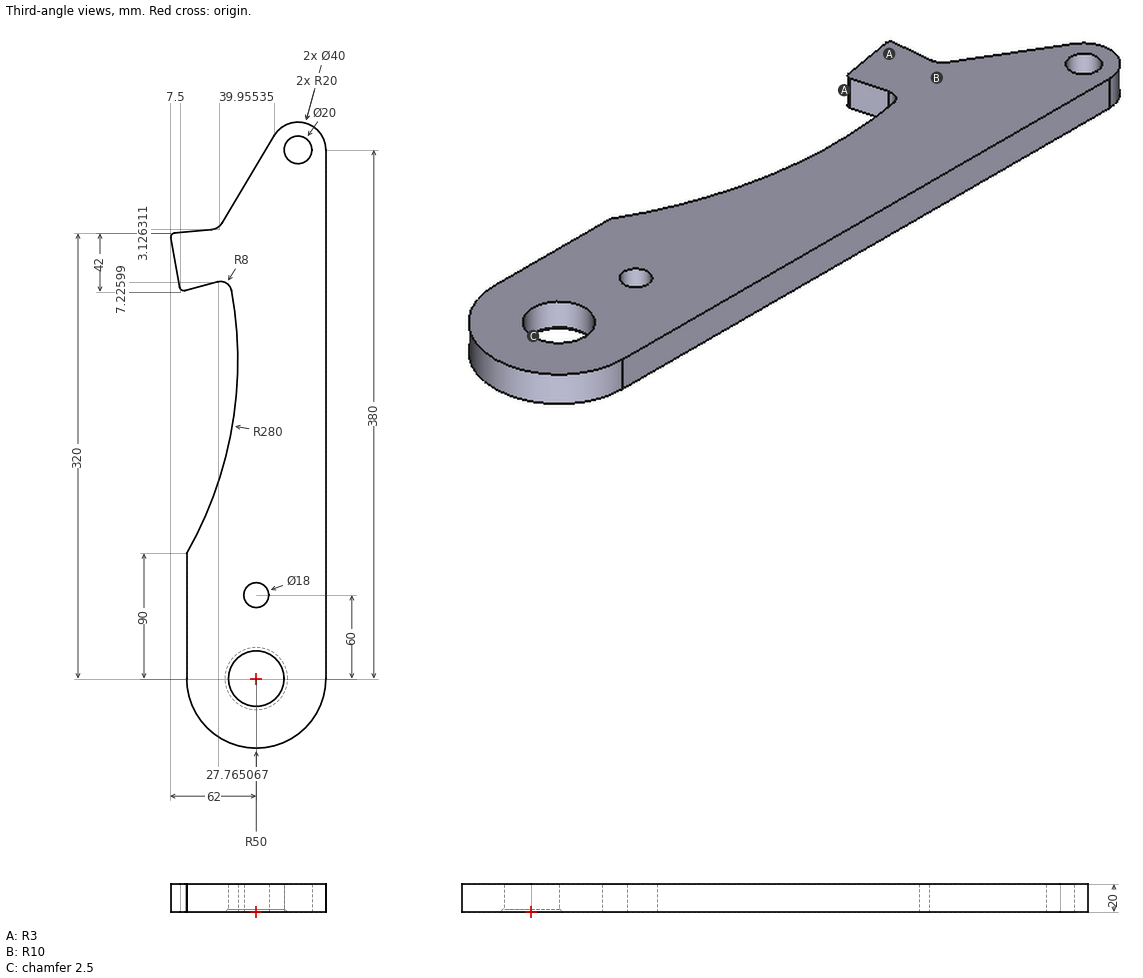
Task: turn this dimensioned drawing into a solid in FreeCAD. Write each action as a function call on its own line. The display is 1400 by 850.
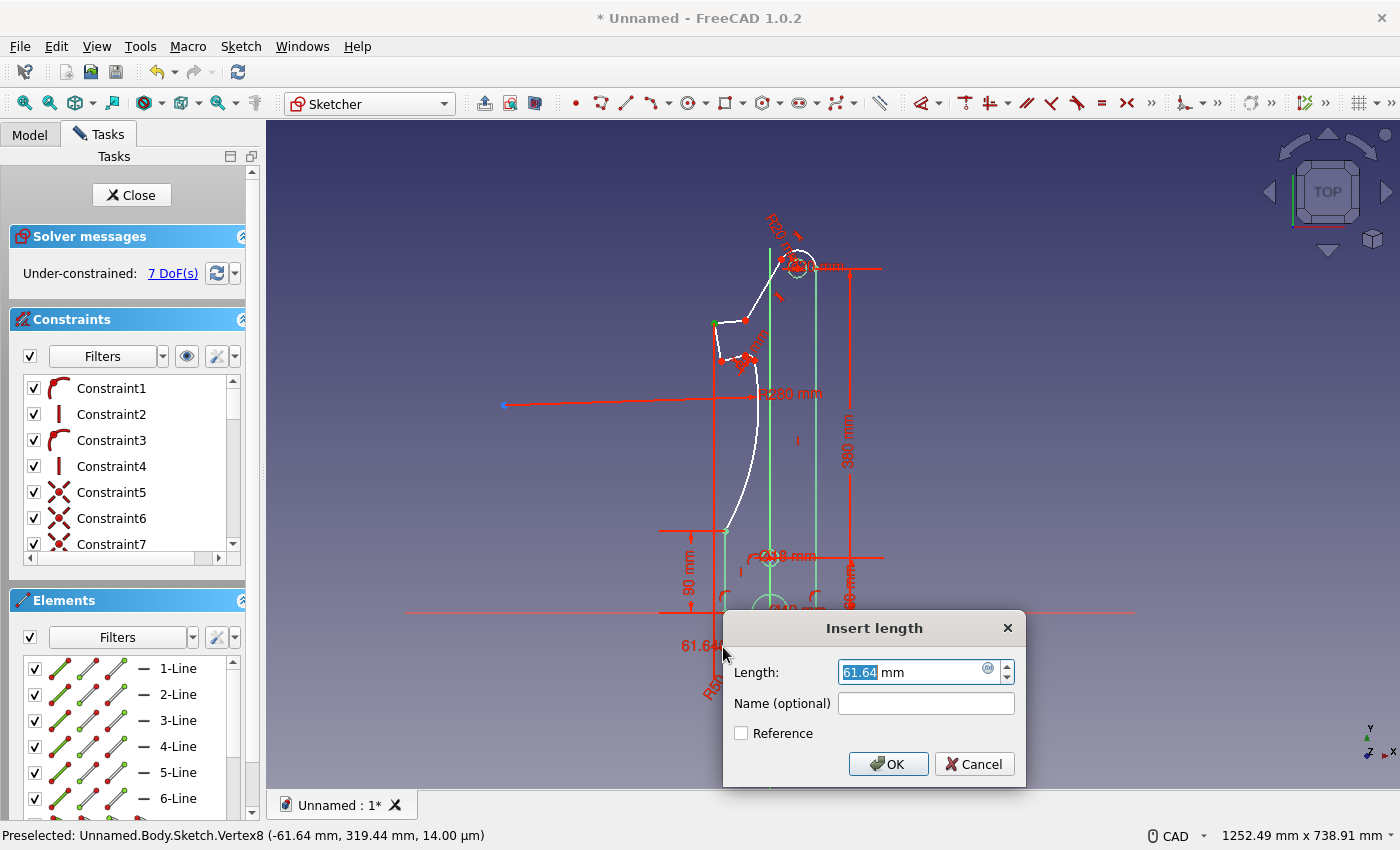
text(62)
key(Return)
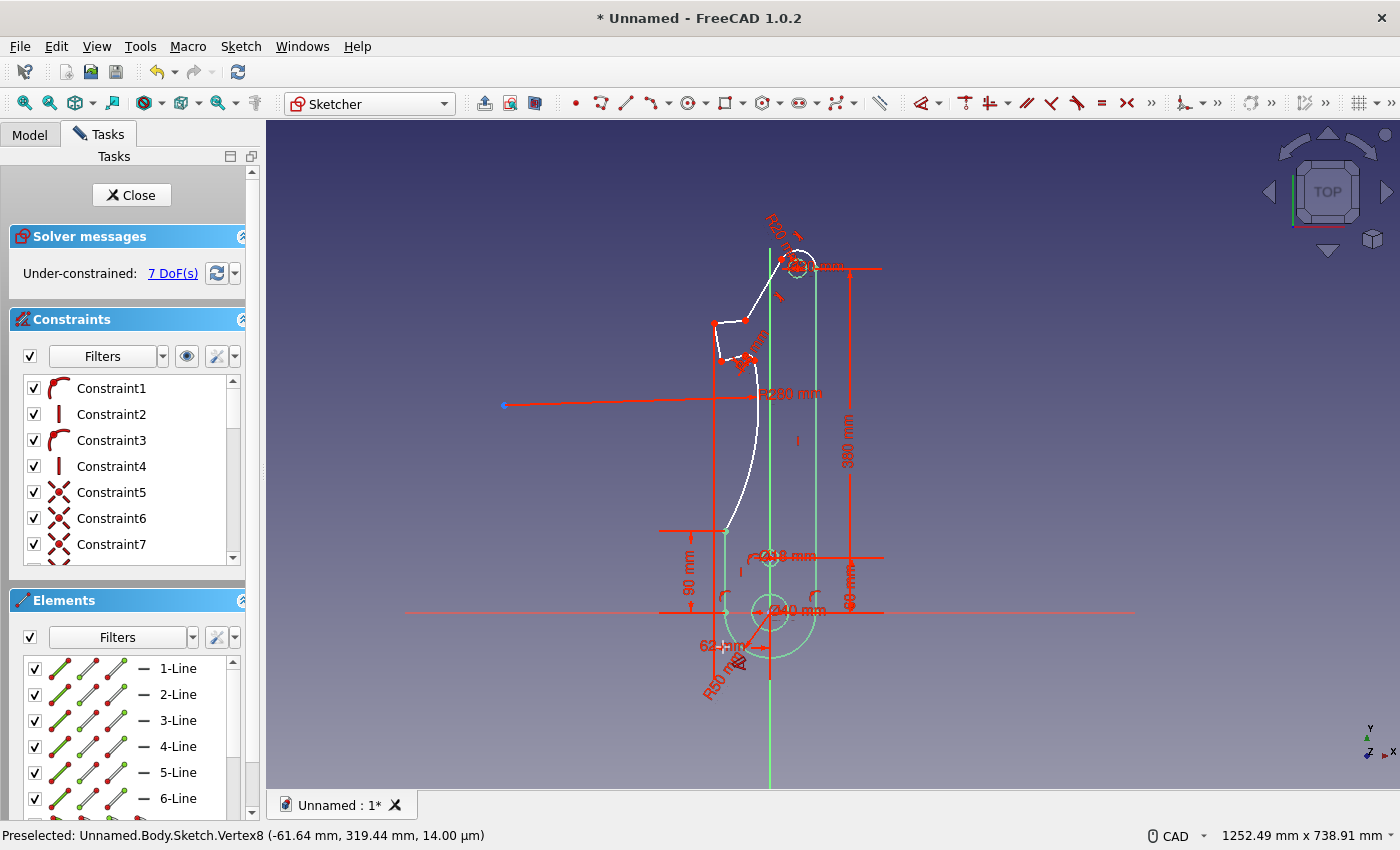
click(716, 335)
click(680, 342)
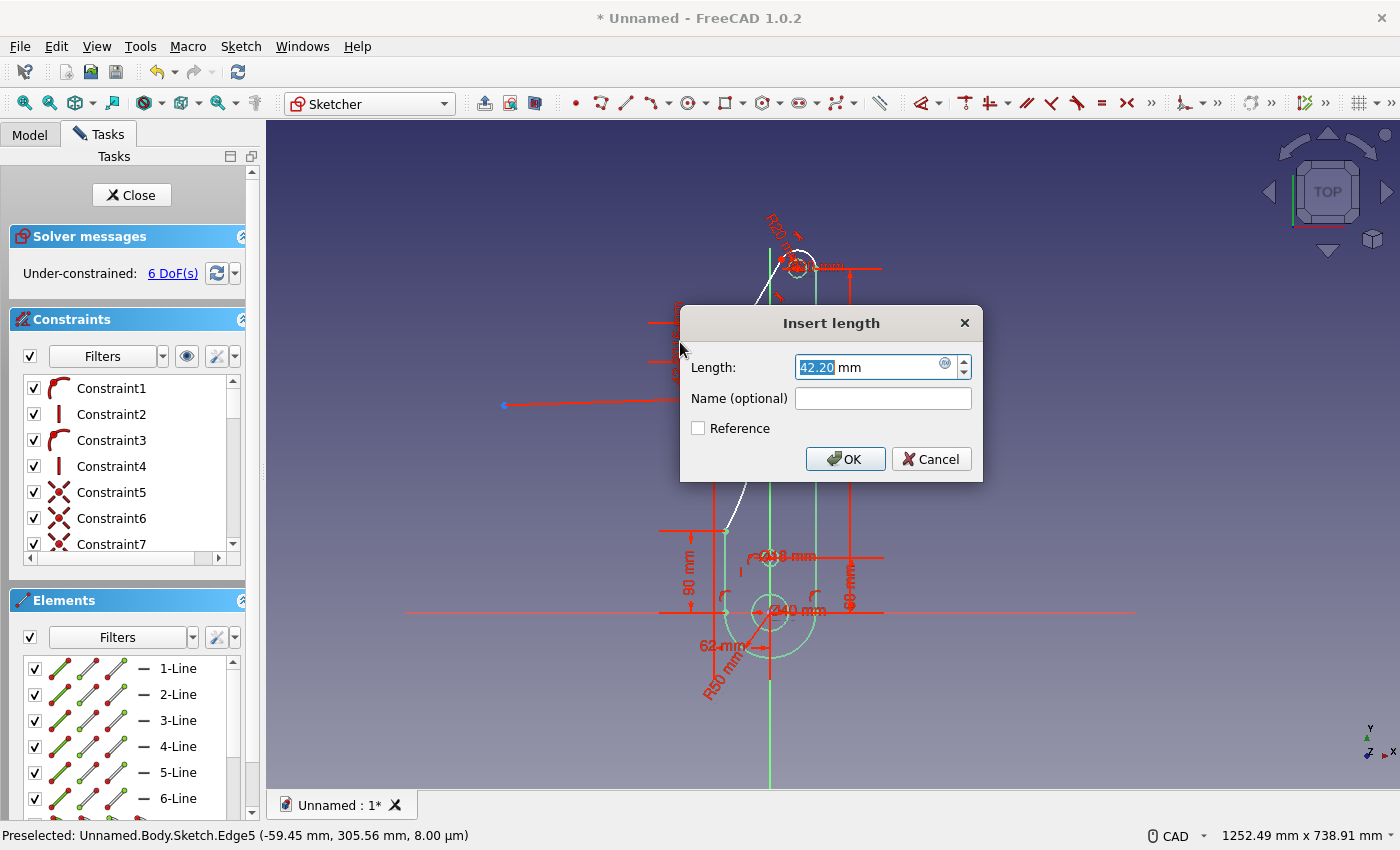
text(42)
key(Return)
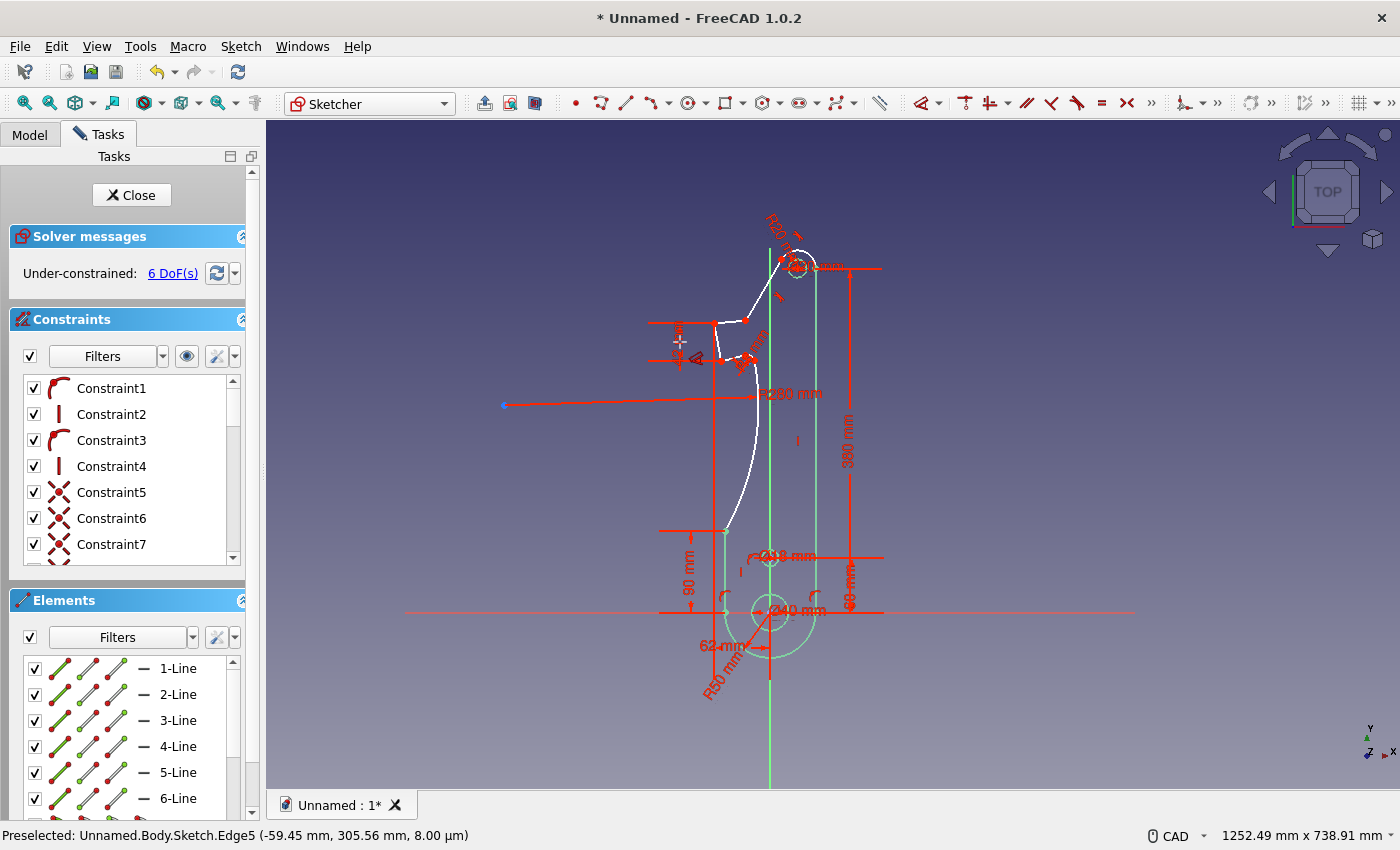
click(714, 323)
click(680, 468)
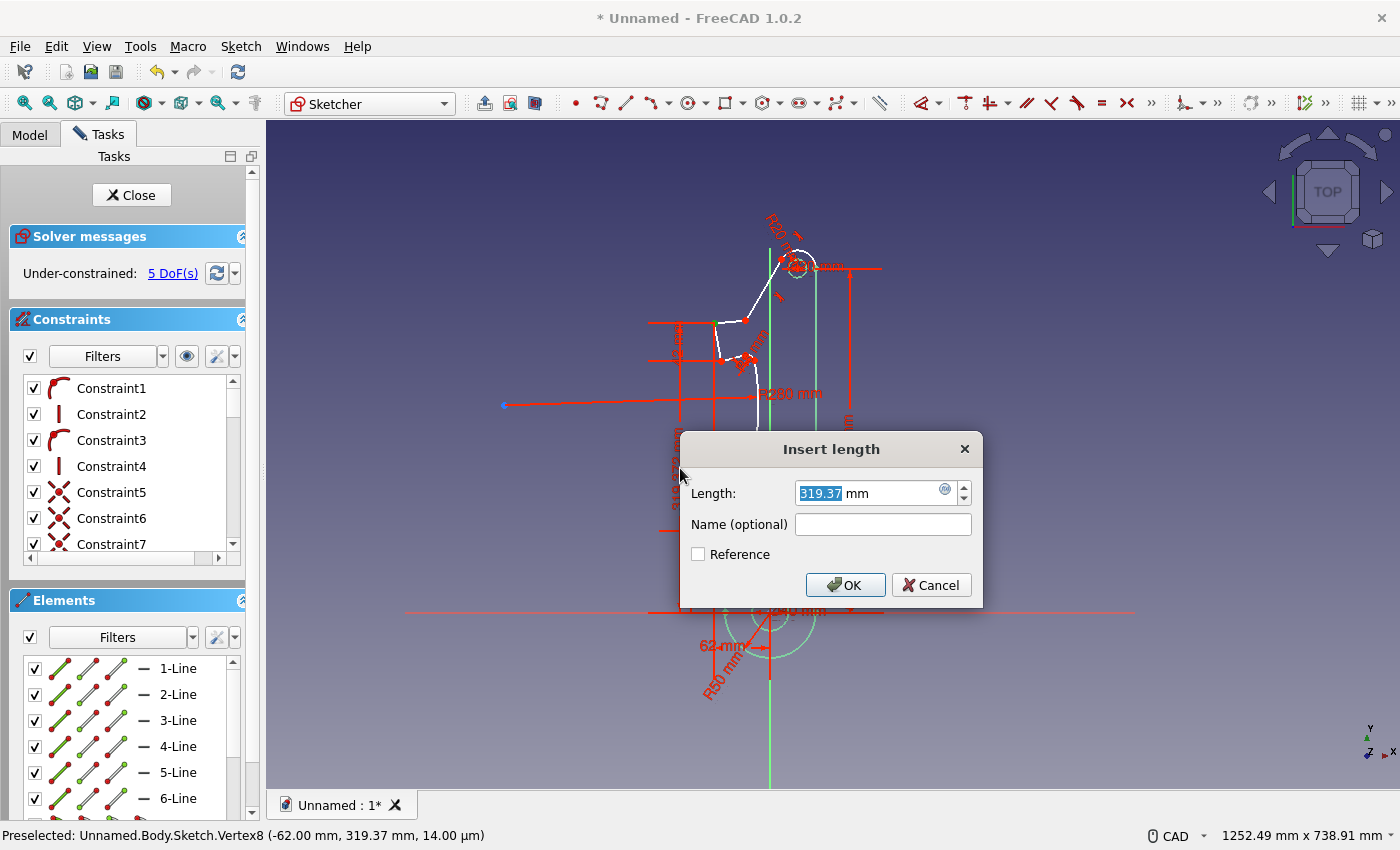
text(320)
key(Return)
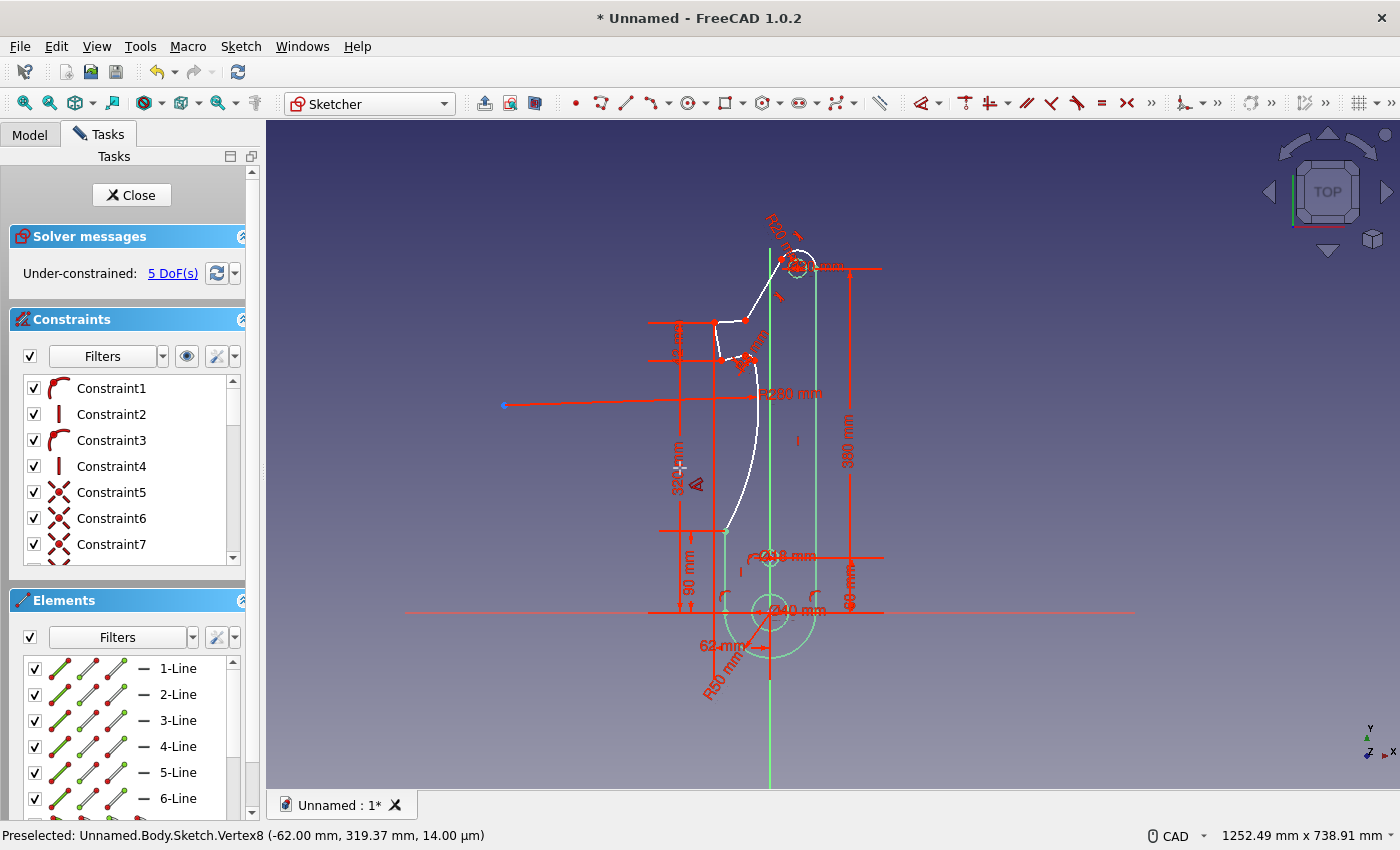
scroll(716, 334, up, 9)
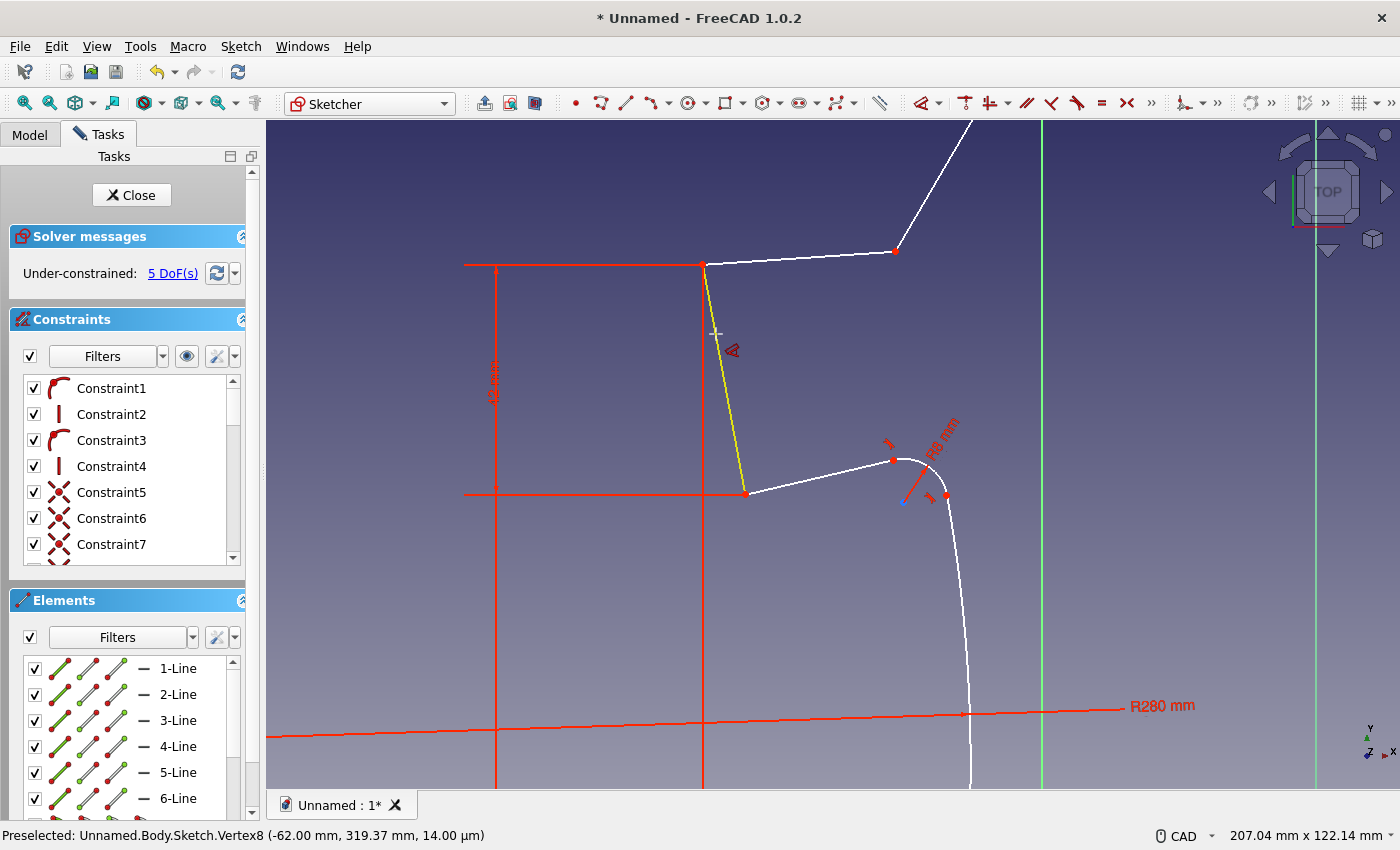
click(716, 334)
click(724, 231)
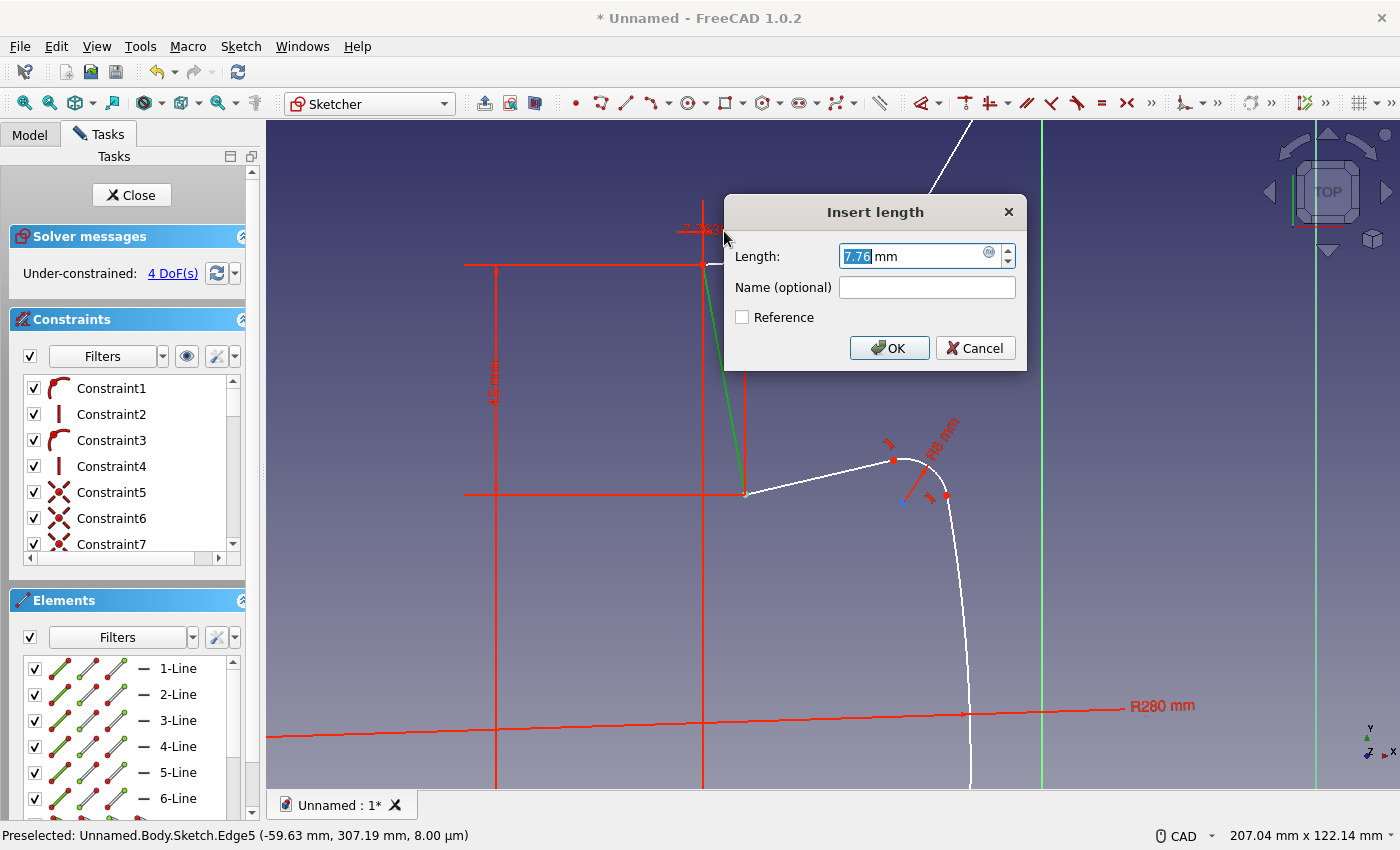
text(7.5)
key(Return)